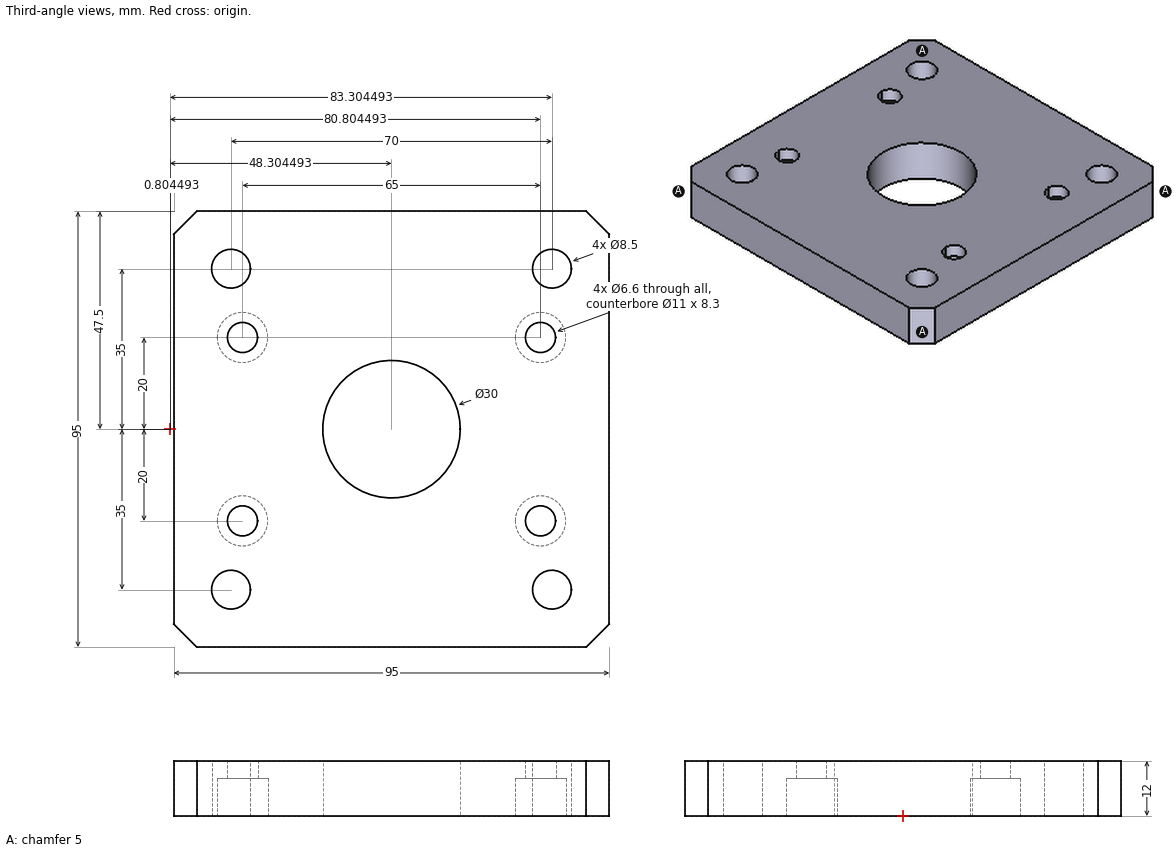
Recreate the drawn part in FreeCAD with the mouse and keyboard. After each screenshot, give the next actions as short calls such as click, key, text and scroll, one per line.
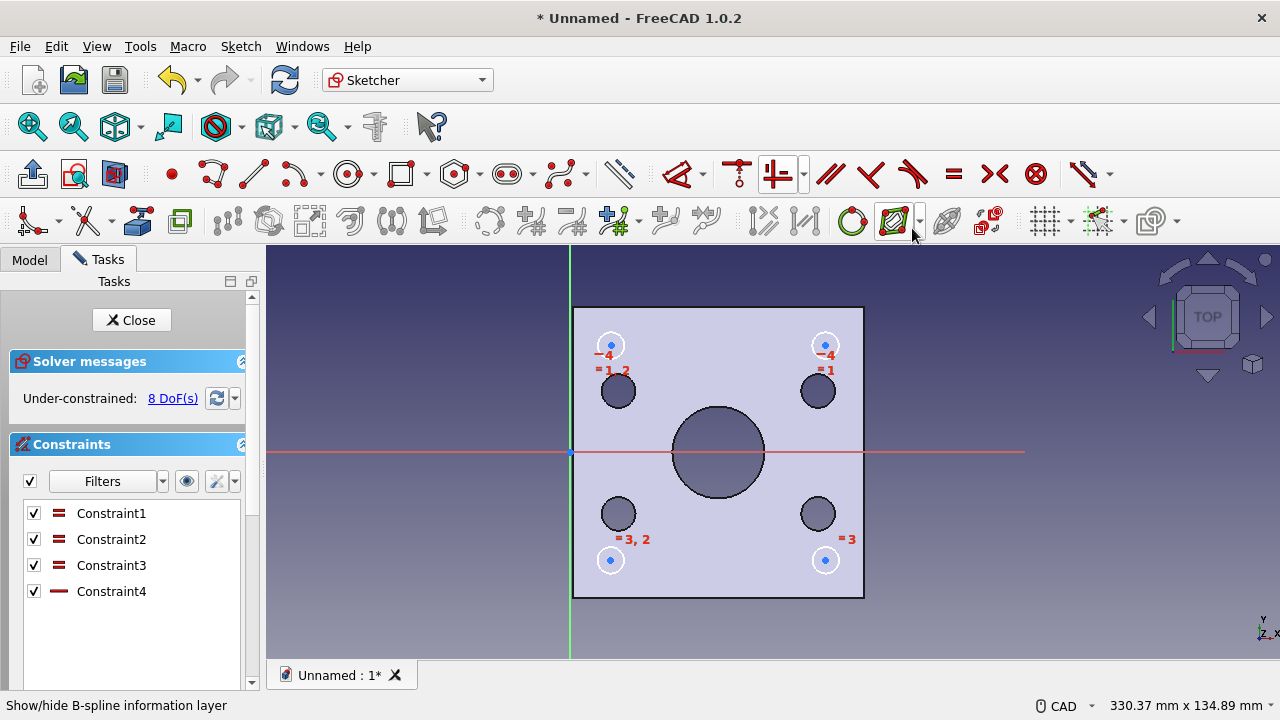
click(611, 346)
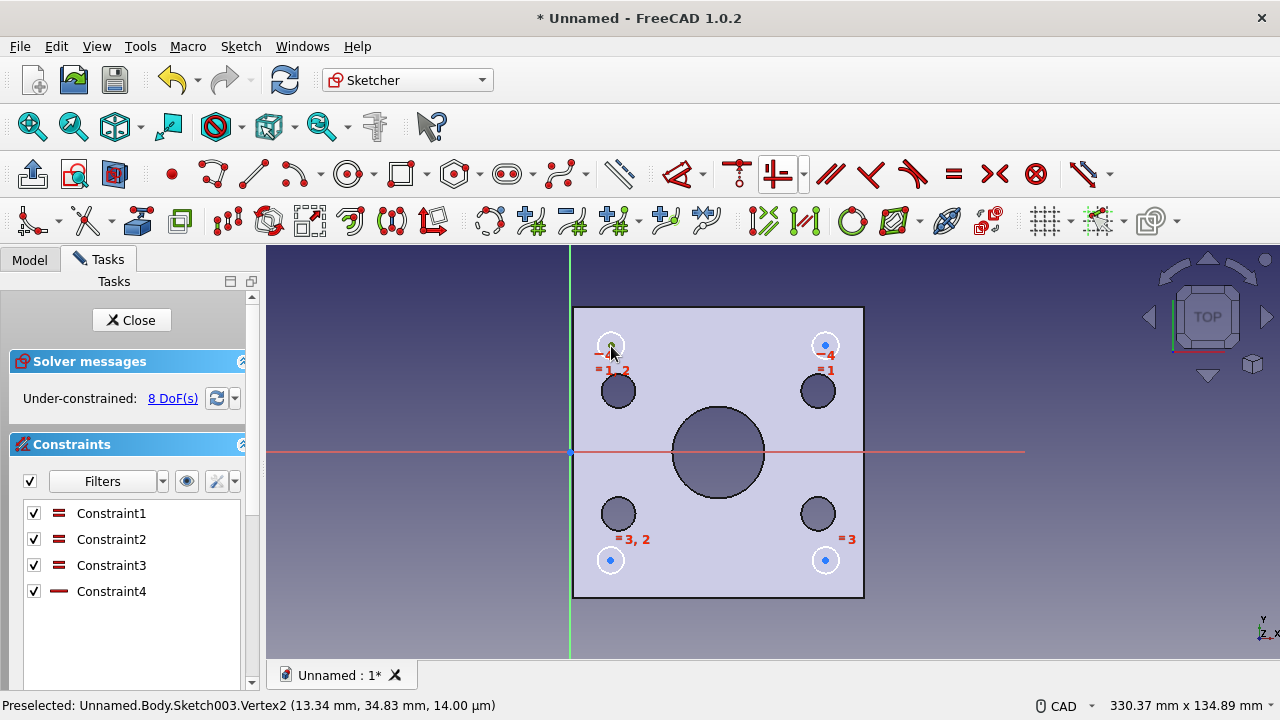
click(611, 560)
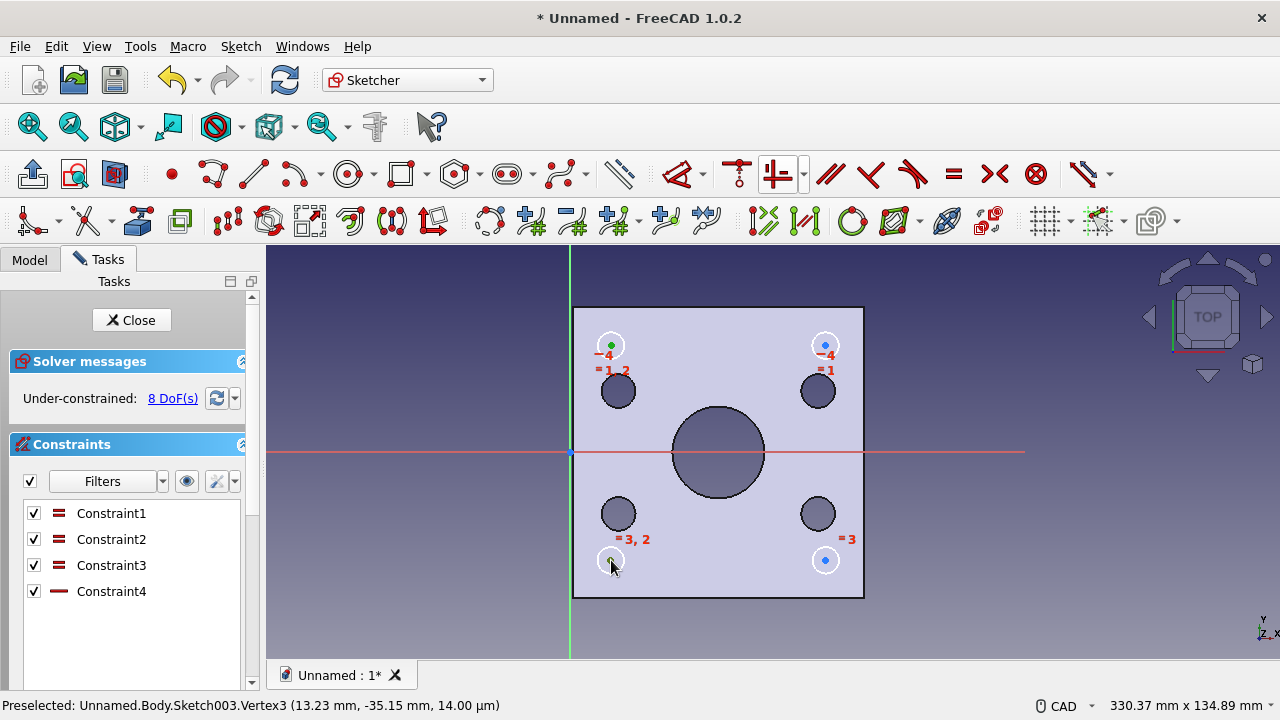
key(v)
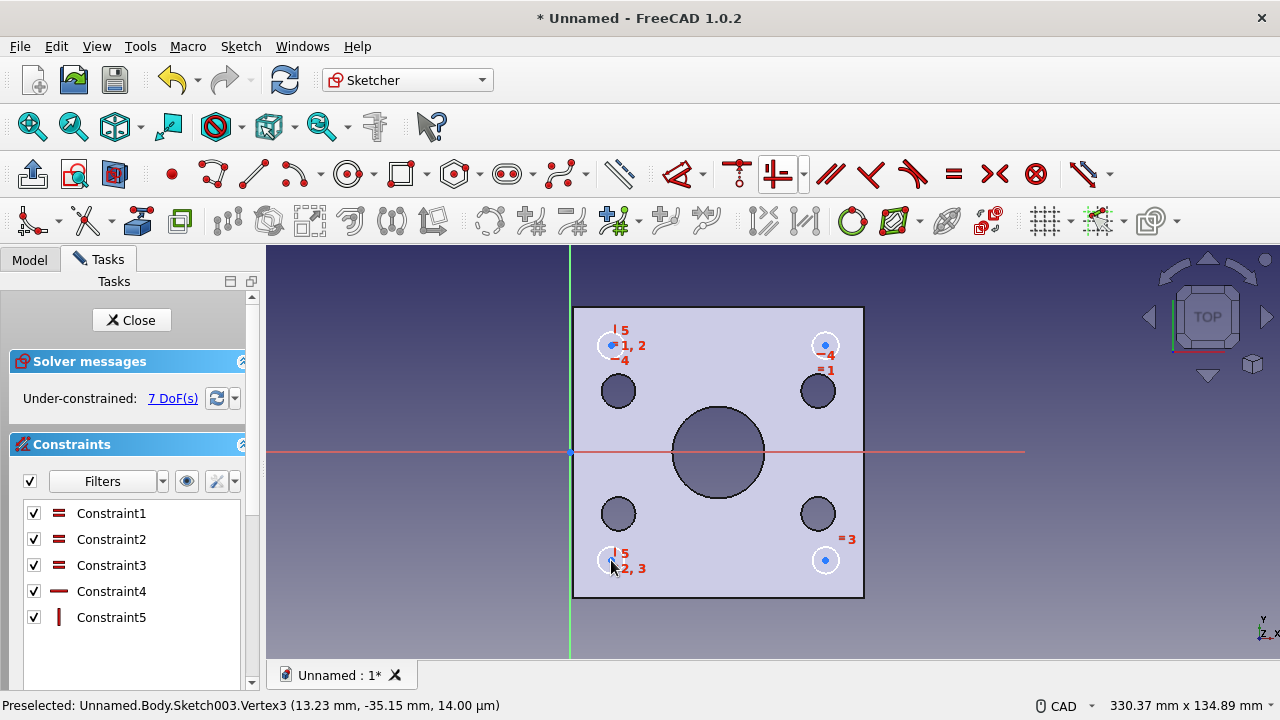
click(826, 346)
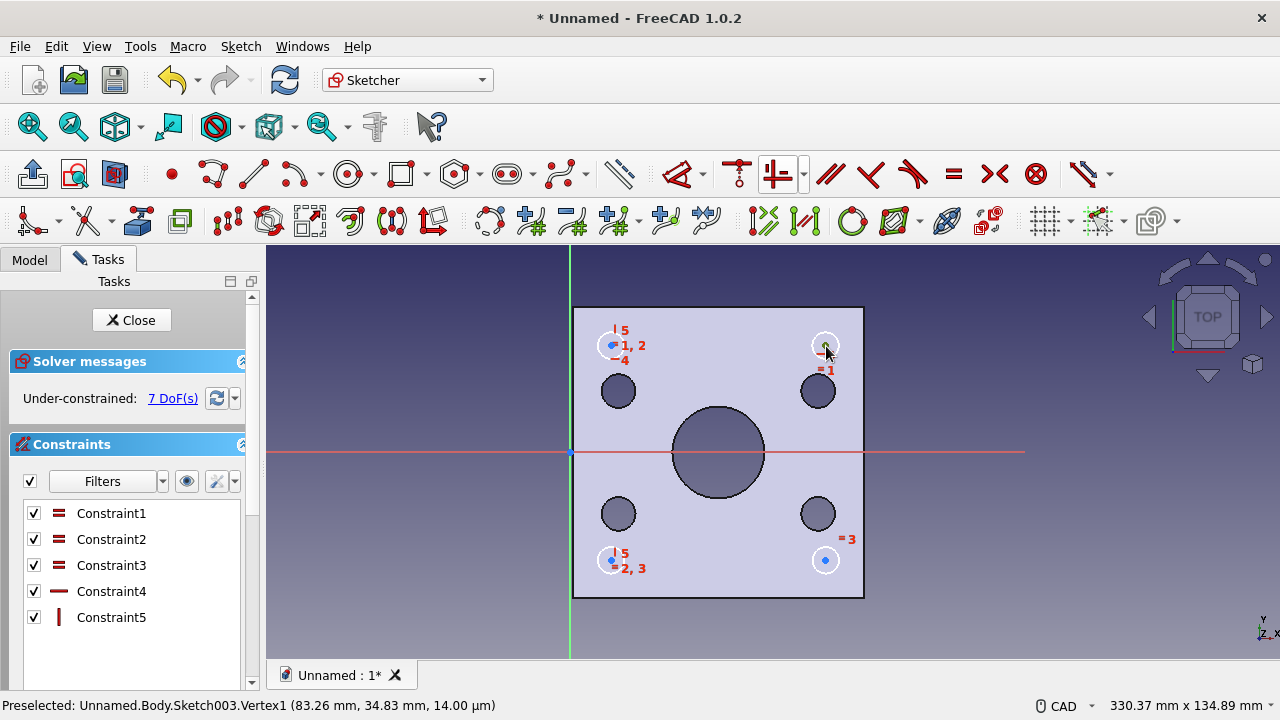
click(826, 560)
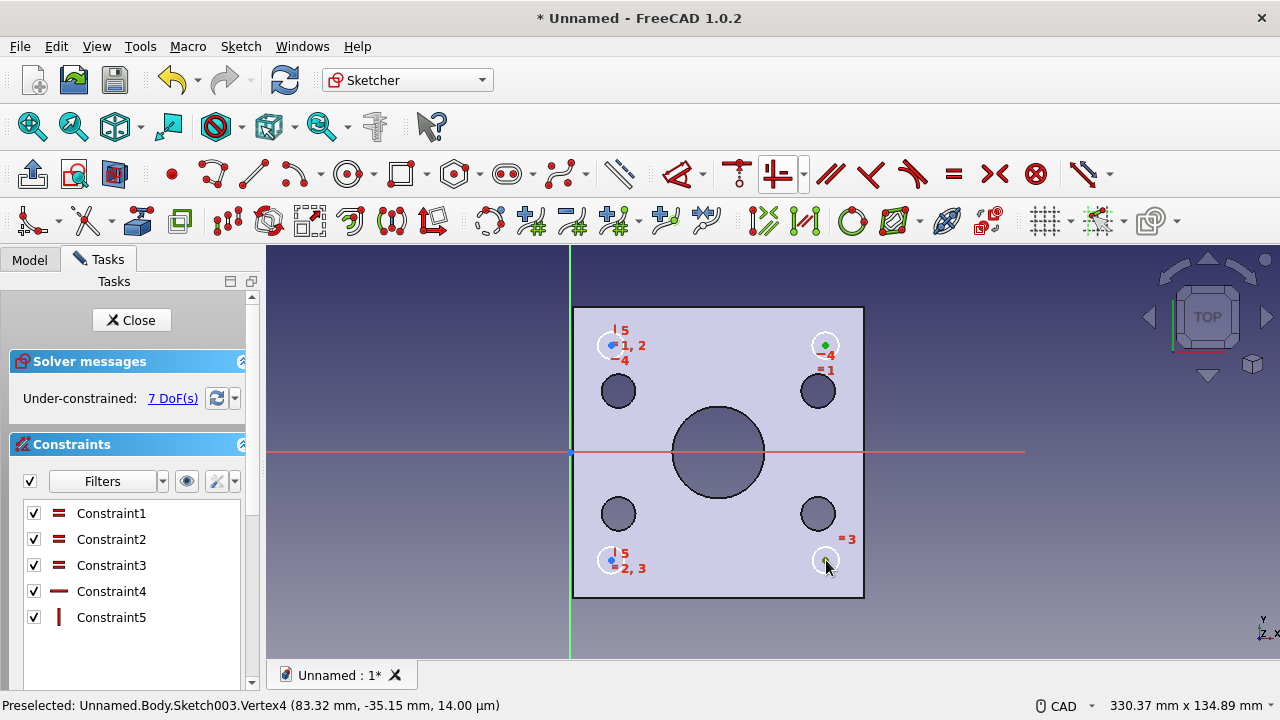
key(v)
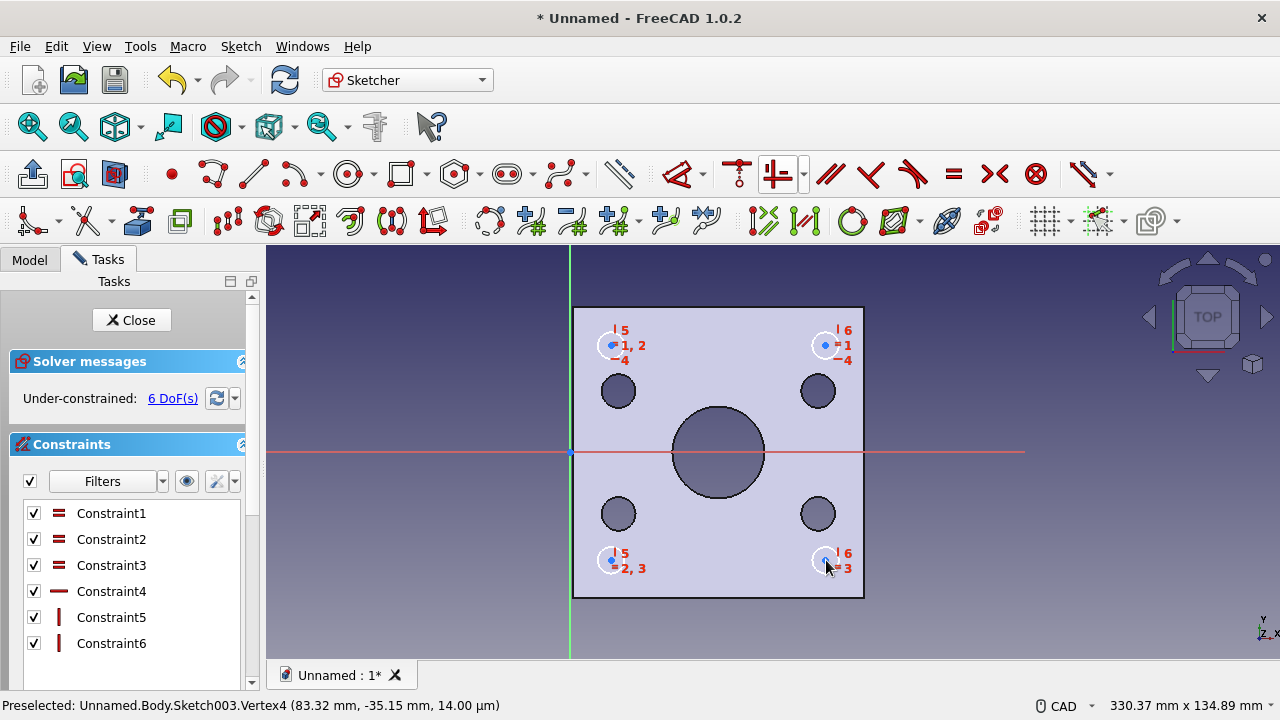
click(609, 562)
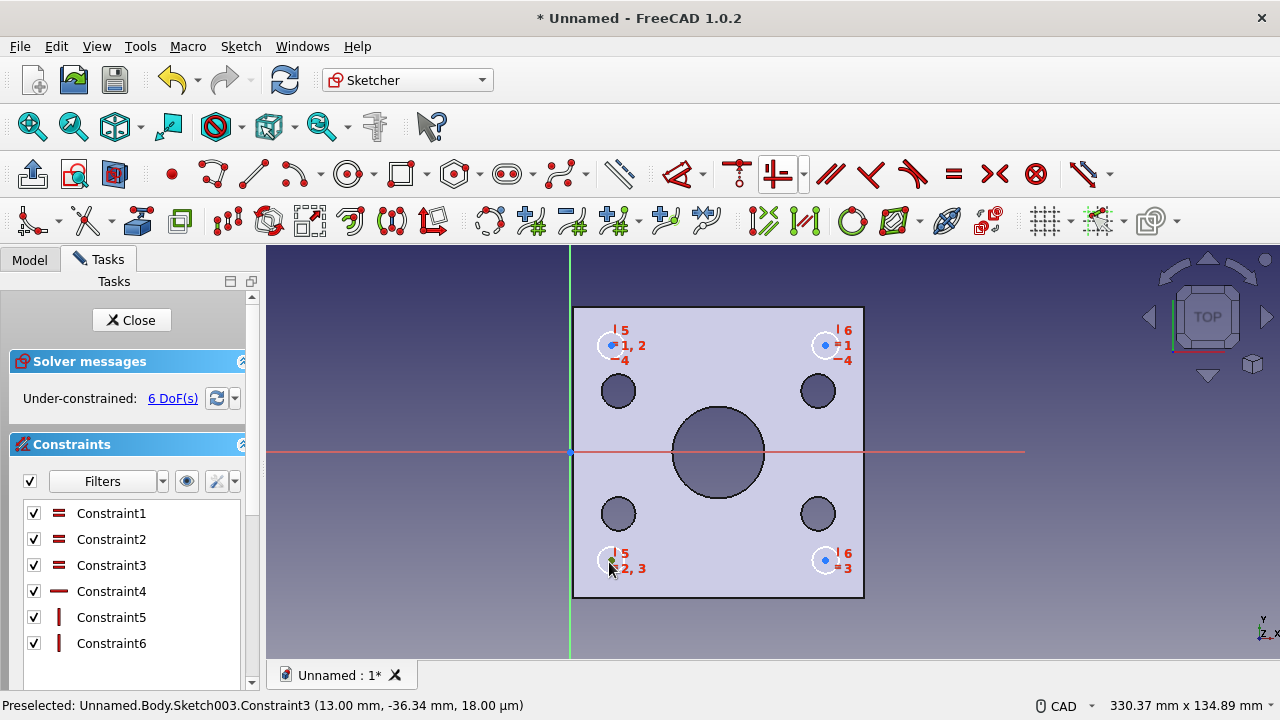
click(826, 560)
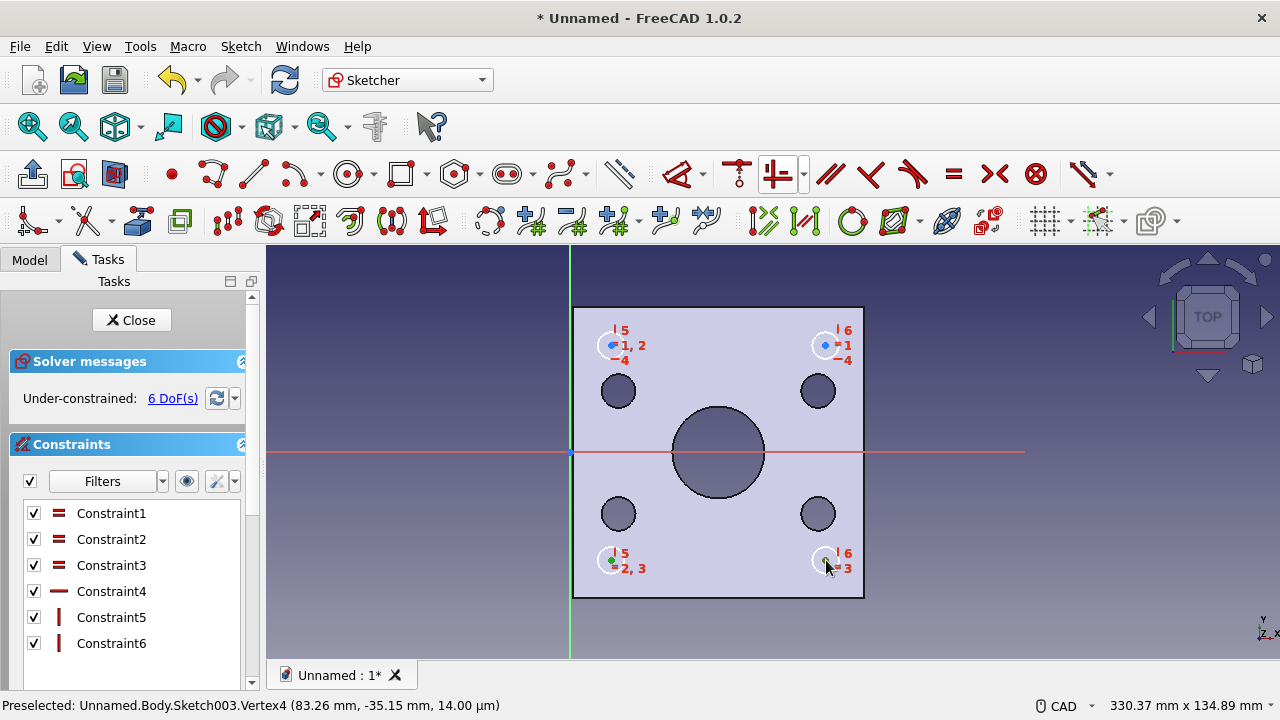
key(h)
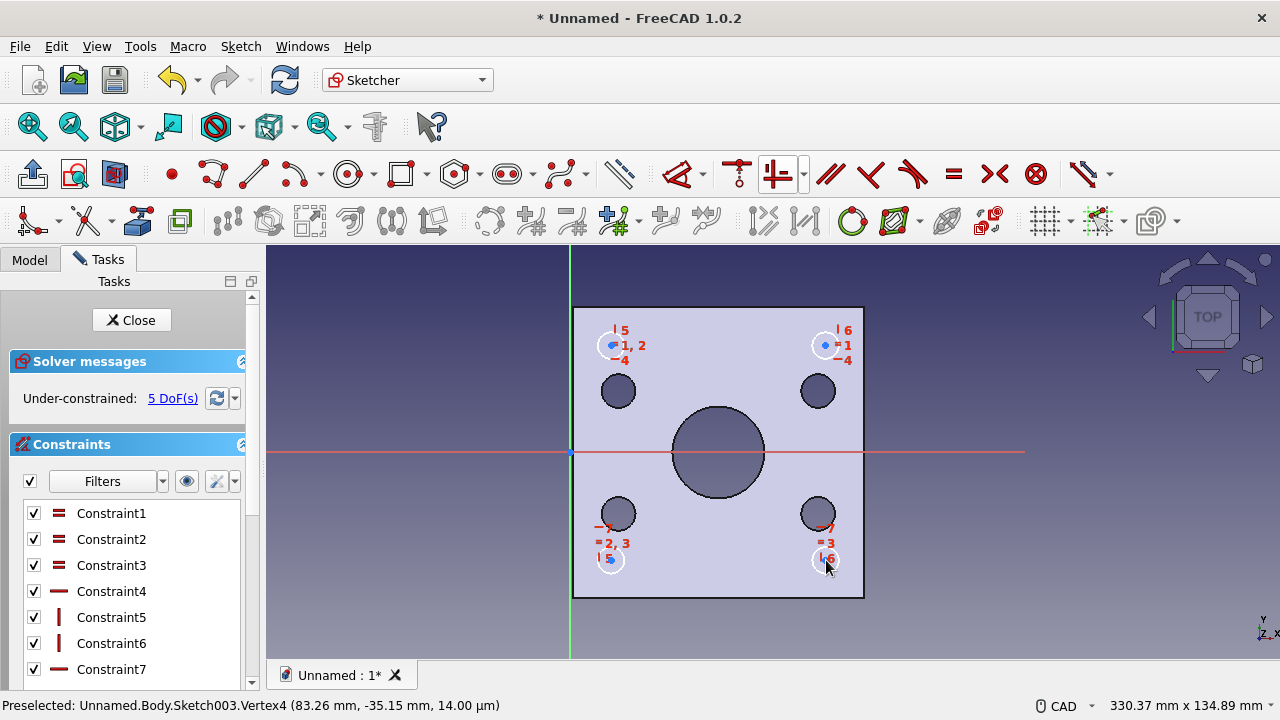
key(d)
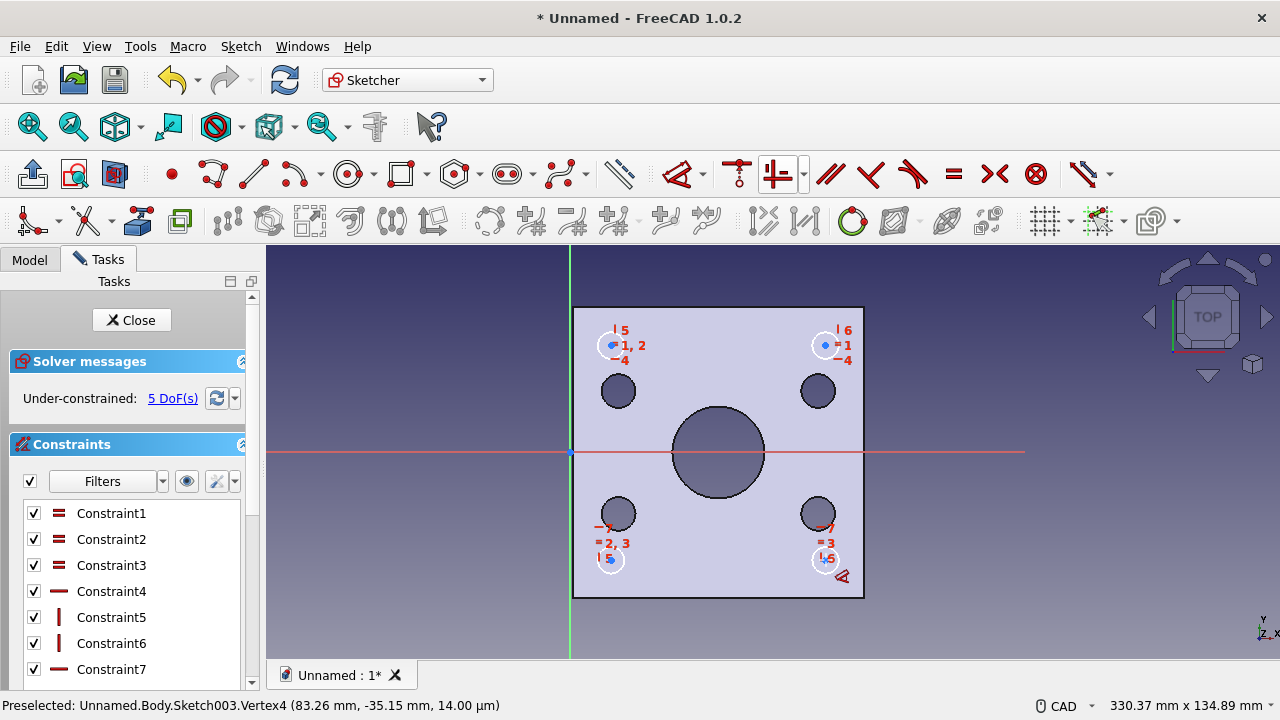
scroll(835, 336, up, 3)